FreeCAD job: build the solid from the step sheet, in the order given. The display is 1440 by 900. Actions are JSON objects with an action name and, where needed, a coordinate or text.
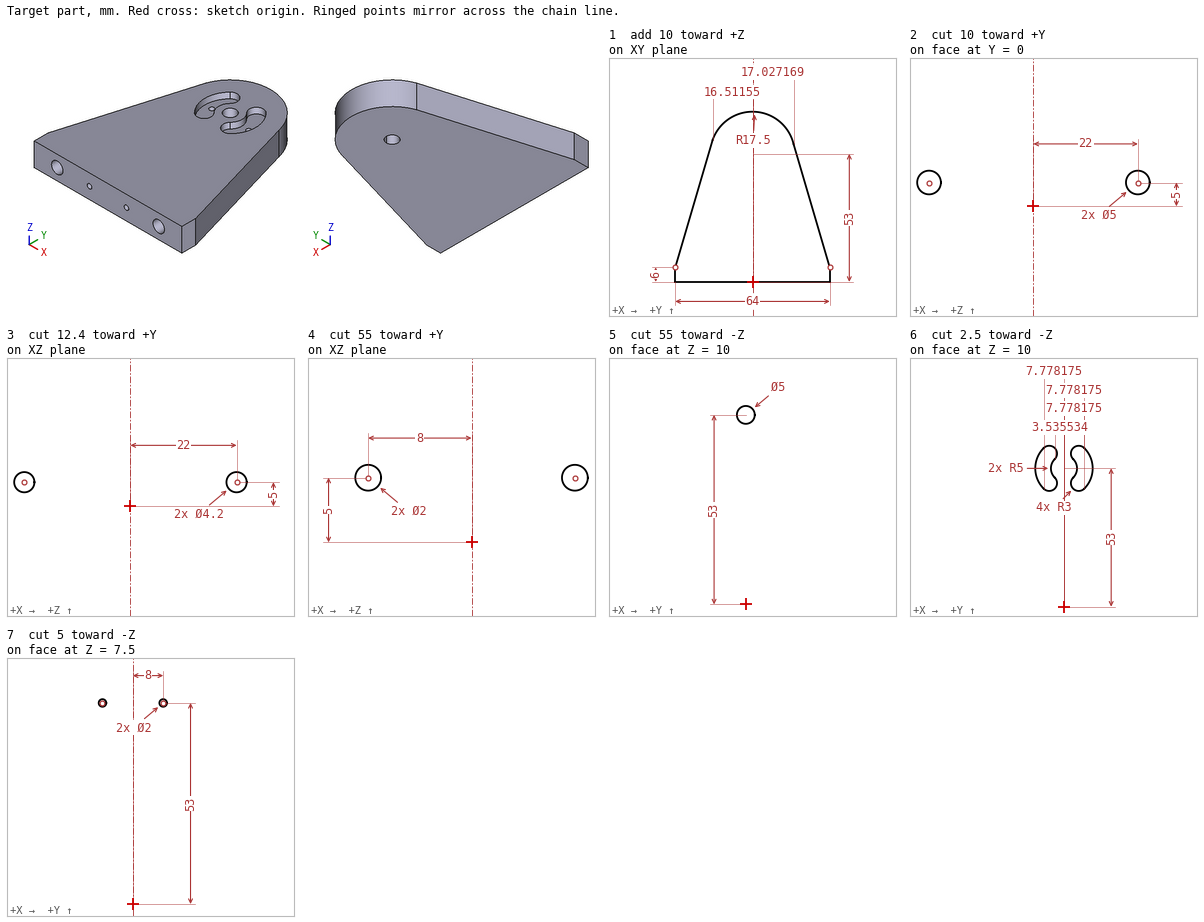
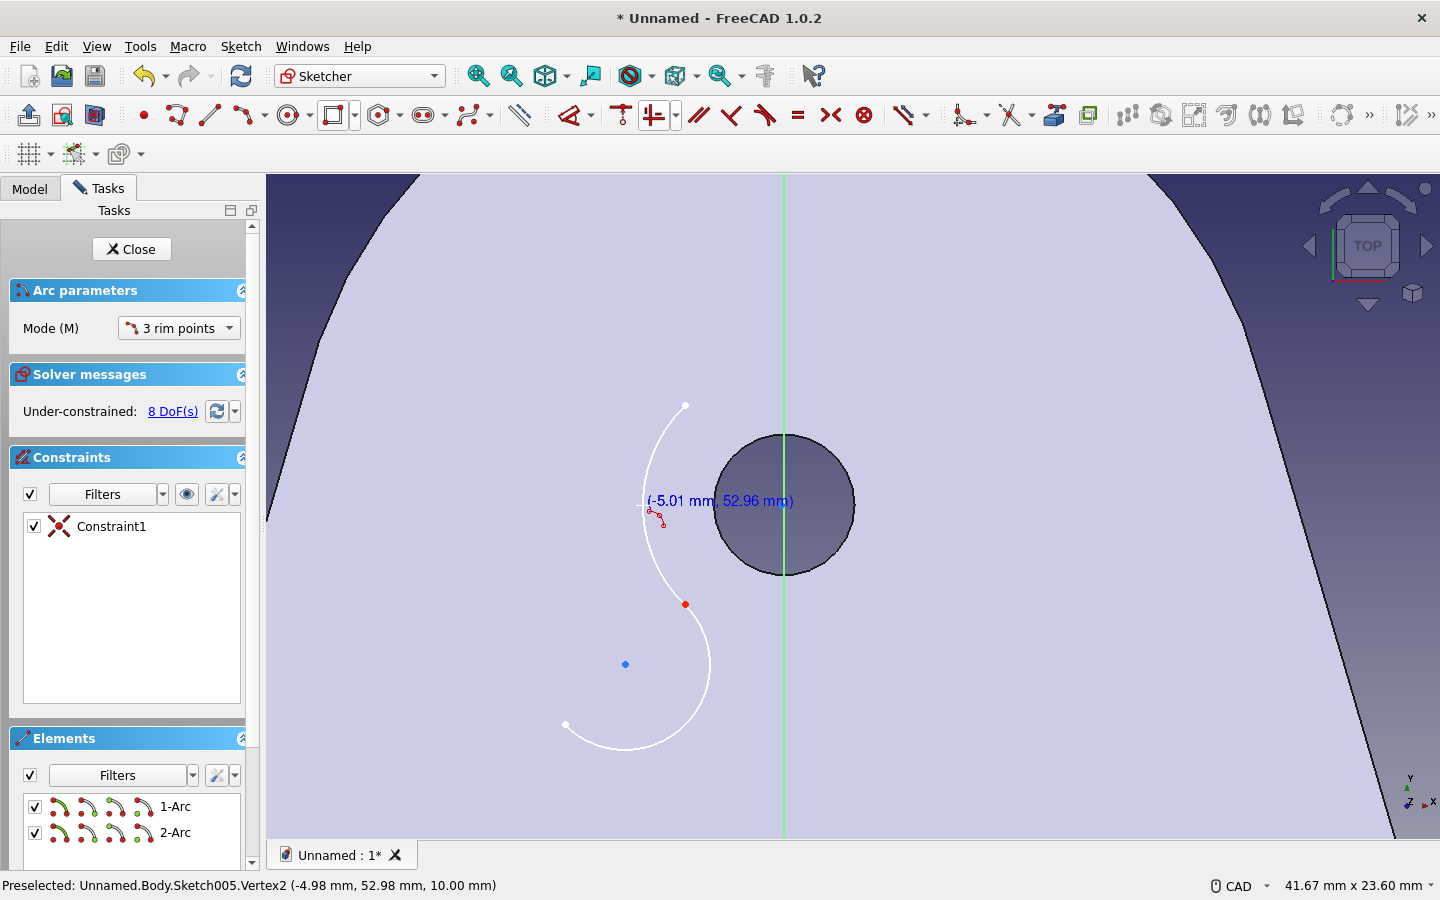
{"action": "left_click", "coordinate": [685, 406]}
{"action": "left_click", "coordinate": [565, 286]}
{"action": "left_click", "coordinate": [685, 286]}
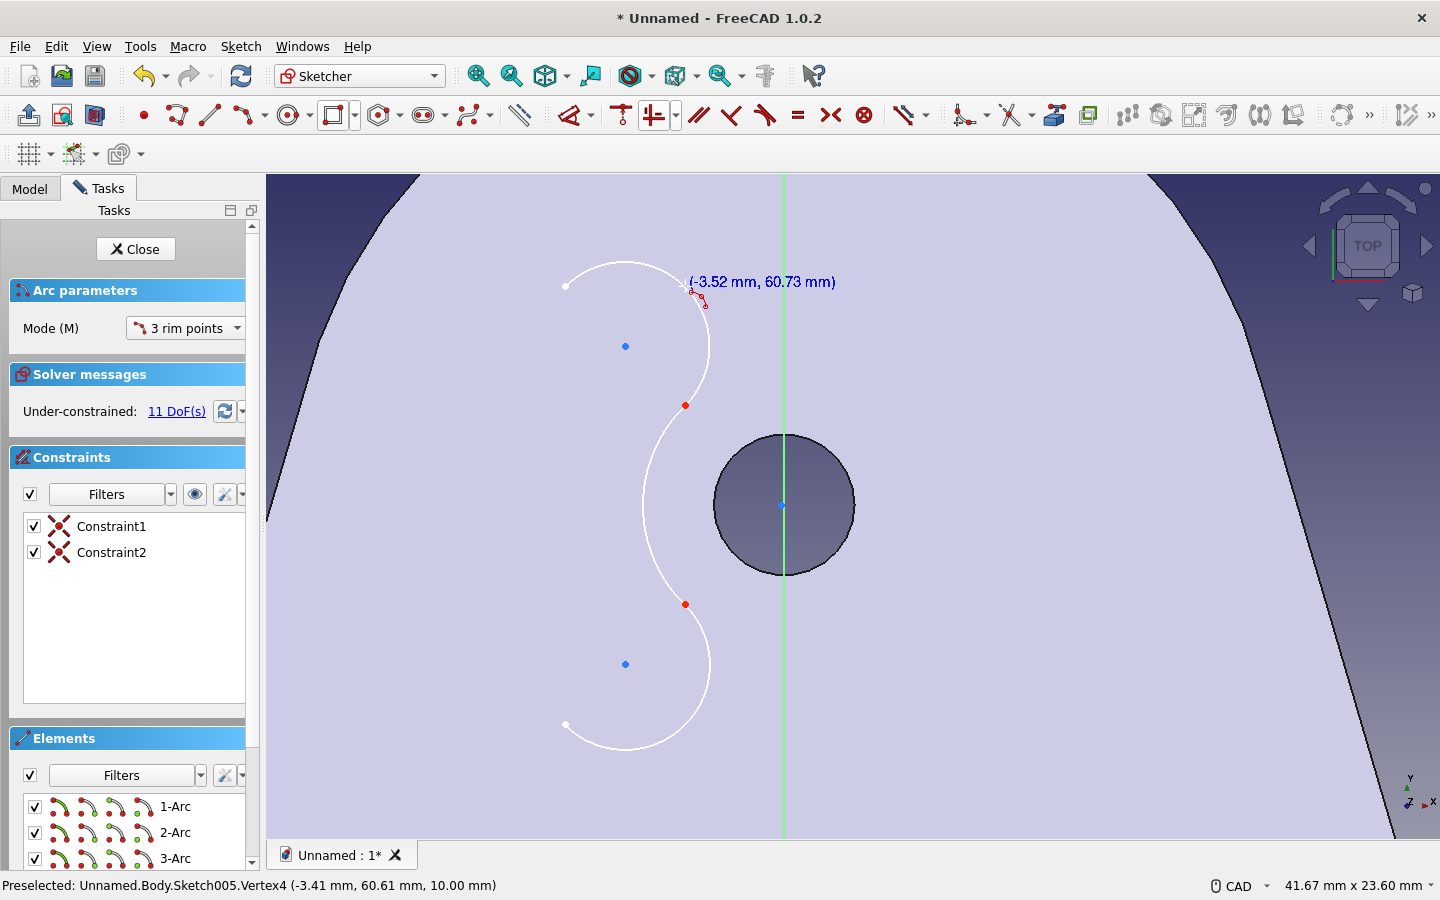
{"action": "left_click", "coordinate": [565, 287]}
{"action": "left_click", "coordinate": [565, 725]}
{"action": "left_click", "coordinate": [474, 505]}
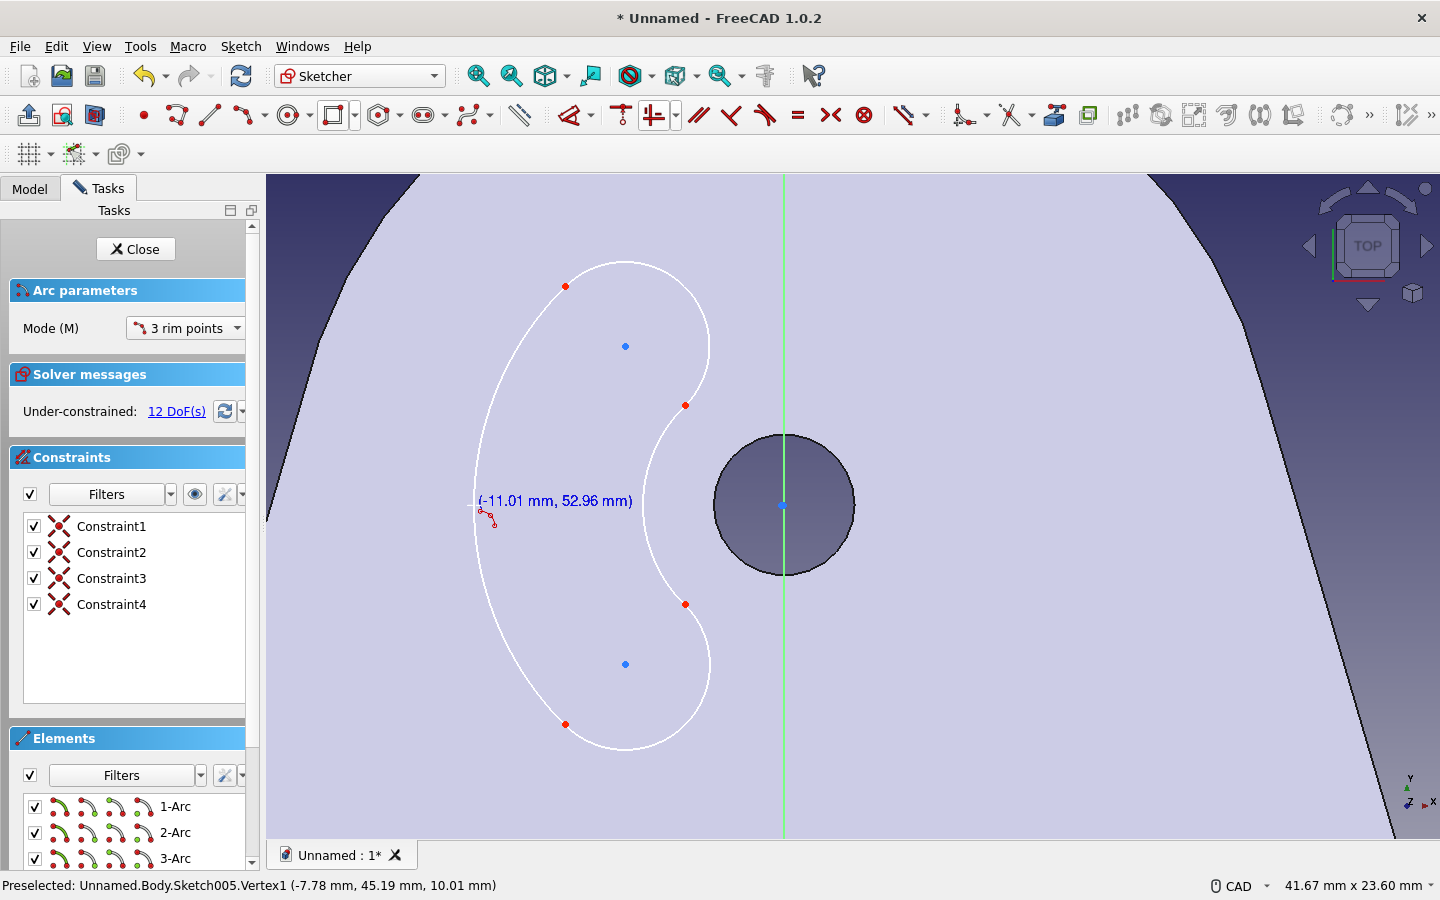
{"action": "left_click", "coordinate": [1003, 724]}
{"action": "left_click", "coordinate": [1003, 286]}
{"action": "left_click", "coordinate": [1094, 505]}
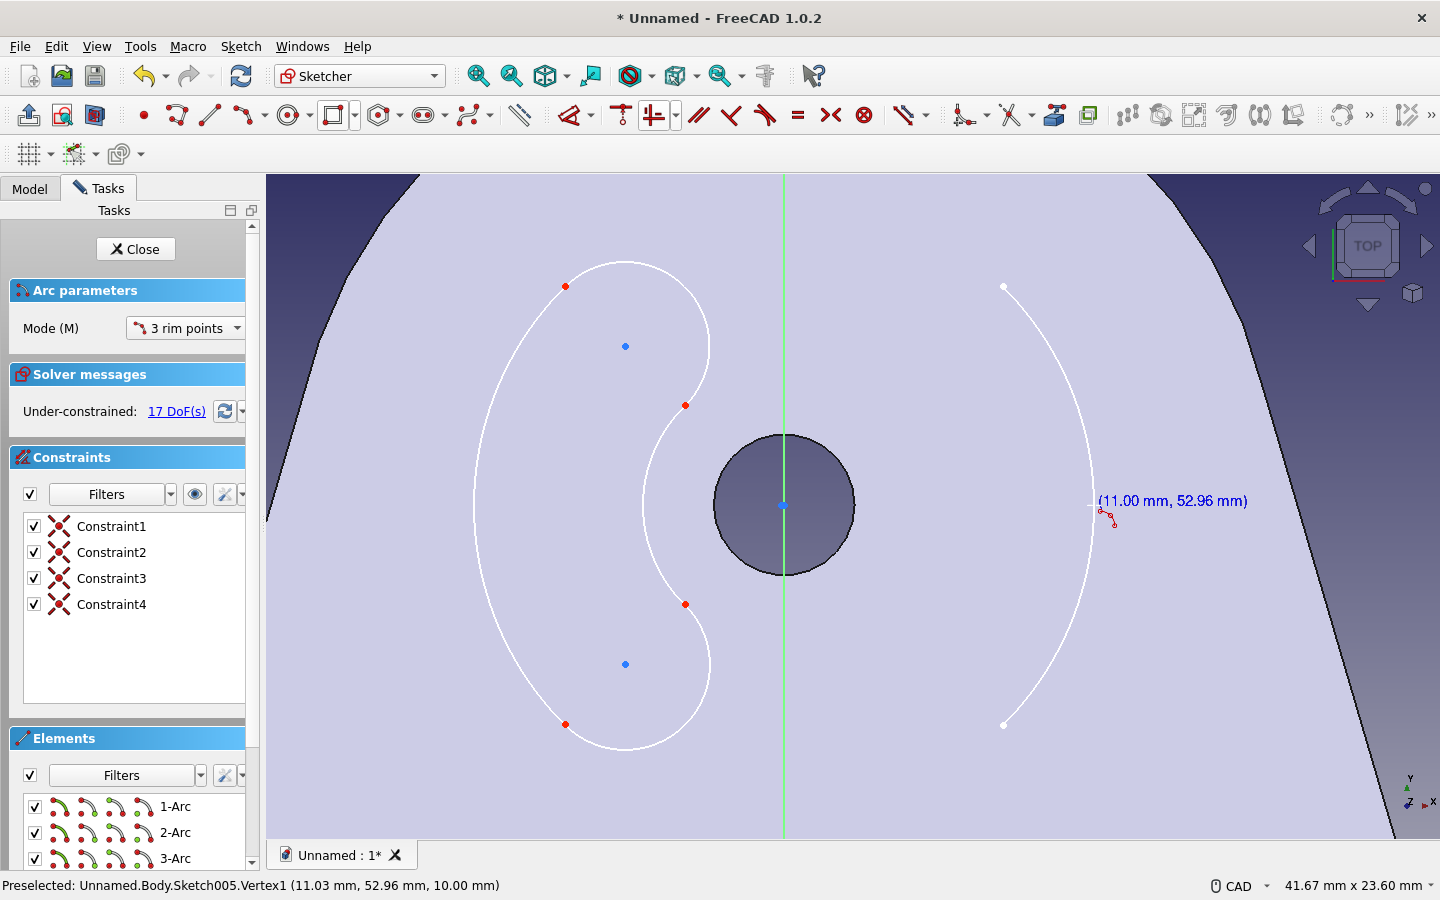
{"action": "left_click", "coordinate": [1003, 287]}
{"action": "left_click", "coordinate": [884, 405]}
{"action": "left_click", "coordinate": [884, 286]}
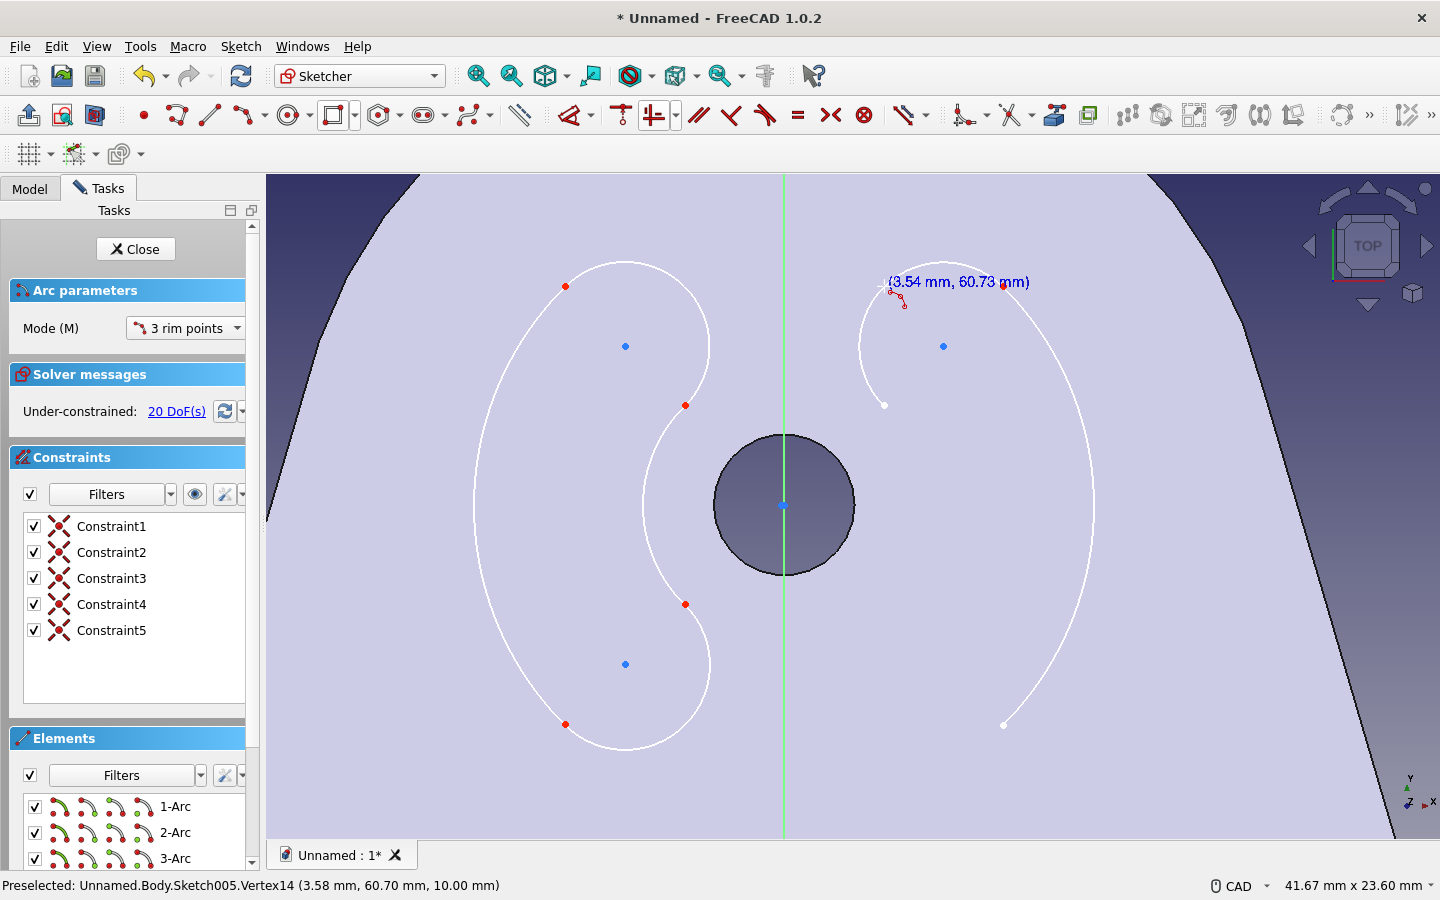
{"action": "left_click", "coordinate": [884, 406]}
{"action": "left_click", "coordinate": [884, 604]}
{"action": "left_click", "coordinate": [925, 505]}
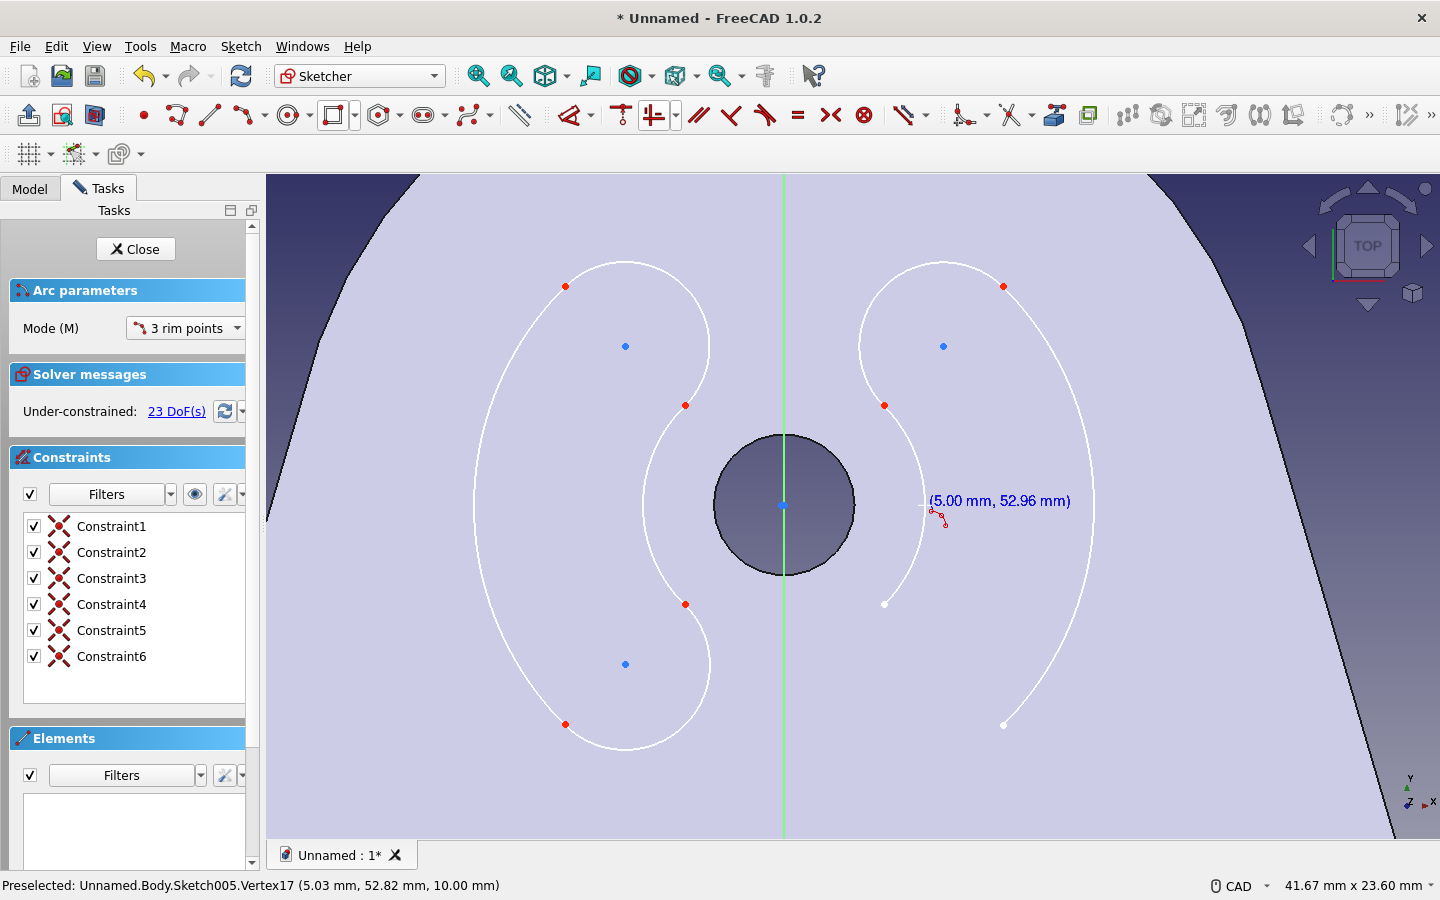
{"action": "left_click", "coordinate": [884, 605]}
{"action": "left_click", "coordinate": [1003, 725]}
{"action": "left_click", "coordinate": [884, 724]}
{"action": "key", "text": "Escape"}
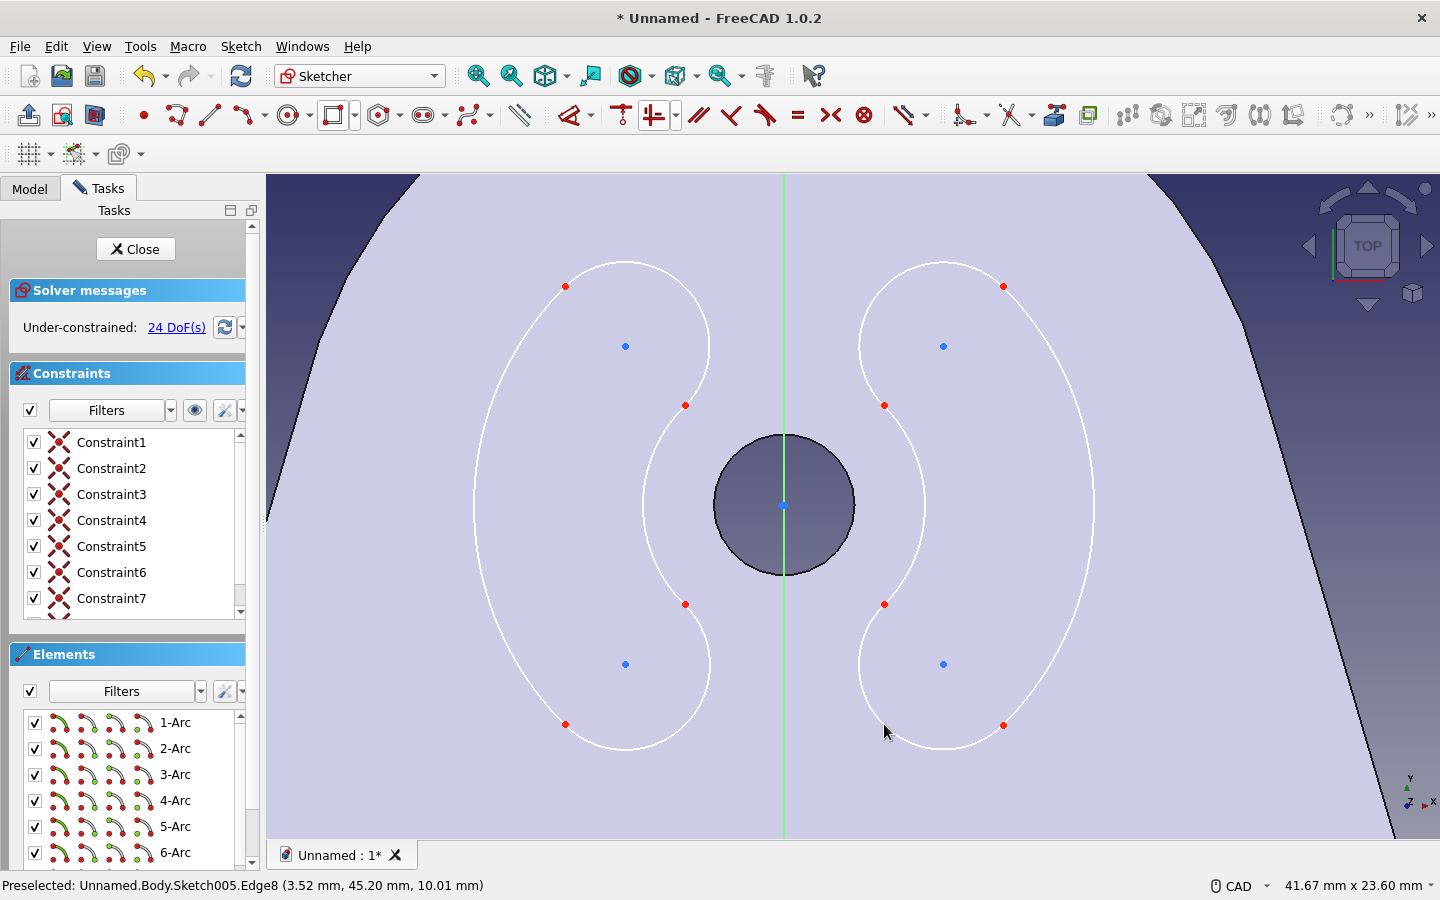
{"action": "left_click", "coordinate": [638, 749]}